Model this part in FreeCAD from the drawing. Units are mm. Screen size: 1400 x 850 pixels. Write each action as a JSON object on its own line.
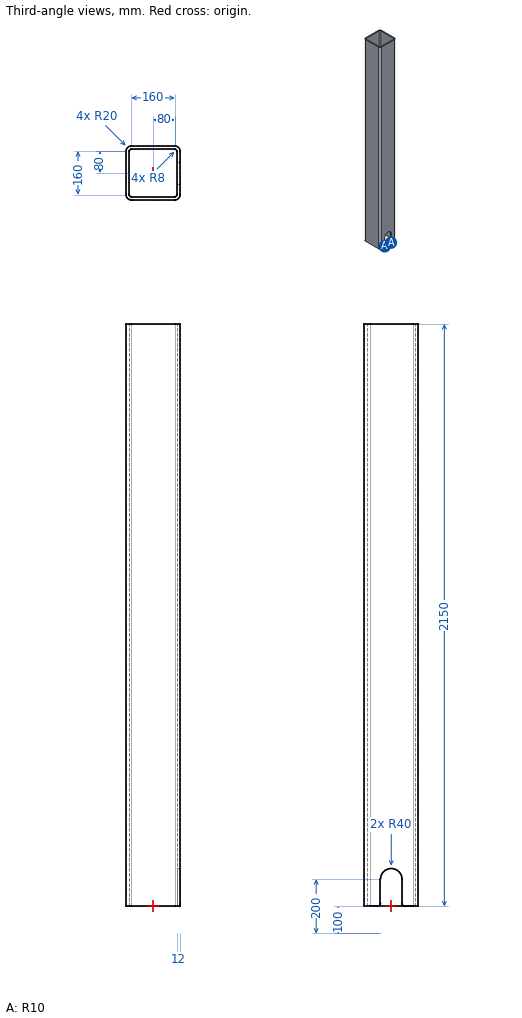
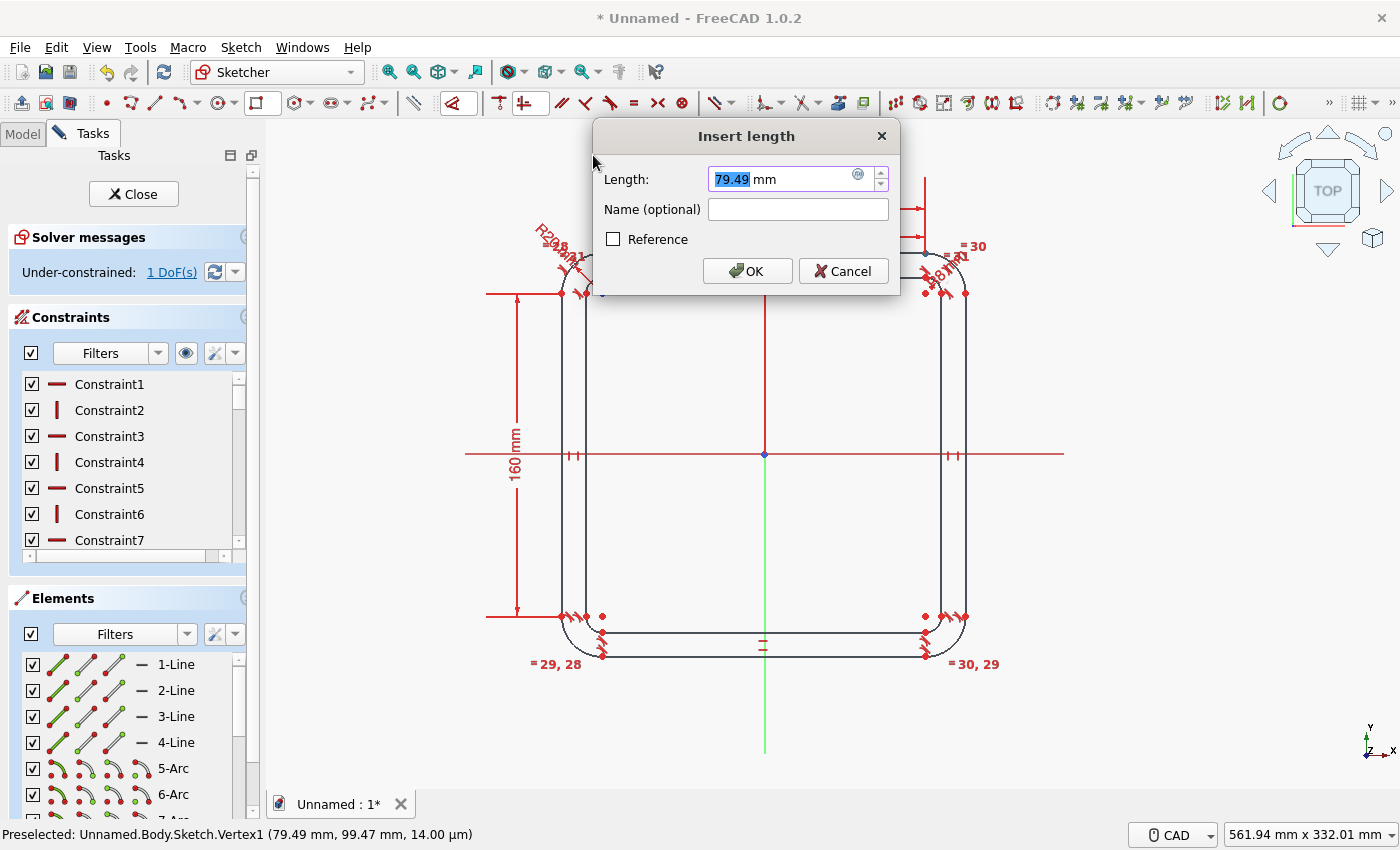
{"action": "type", "text": "80"}
{"action": "key", "text": "Return"}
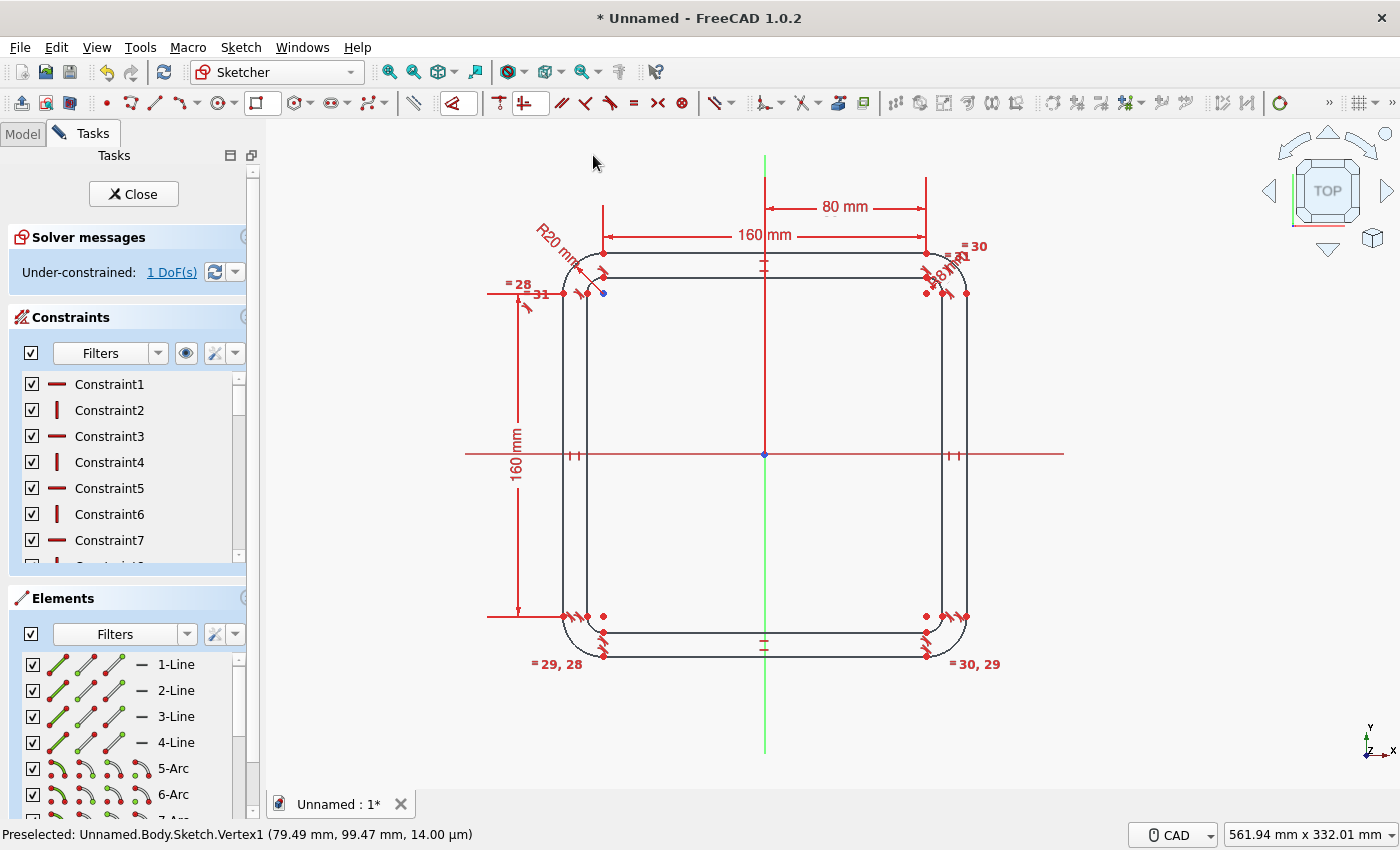
{"action": "left_click", "coordinate": [563, 294]}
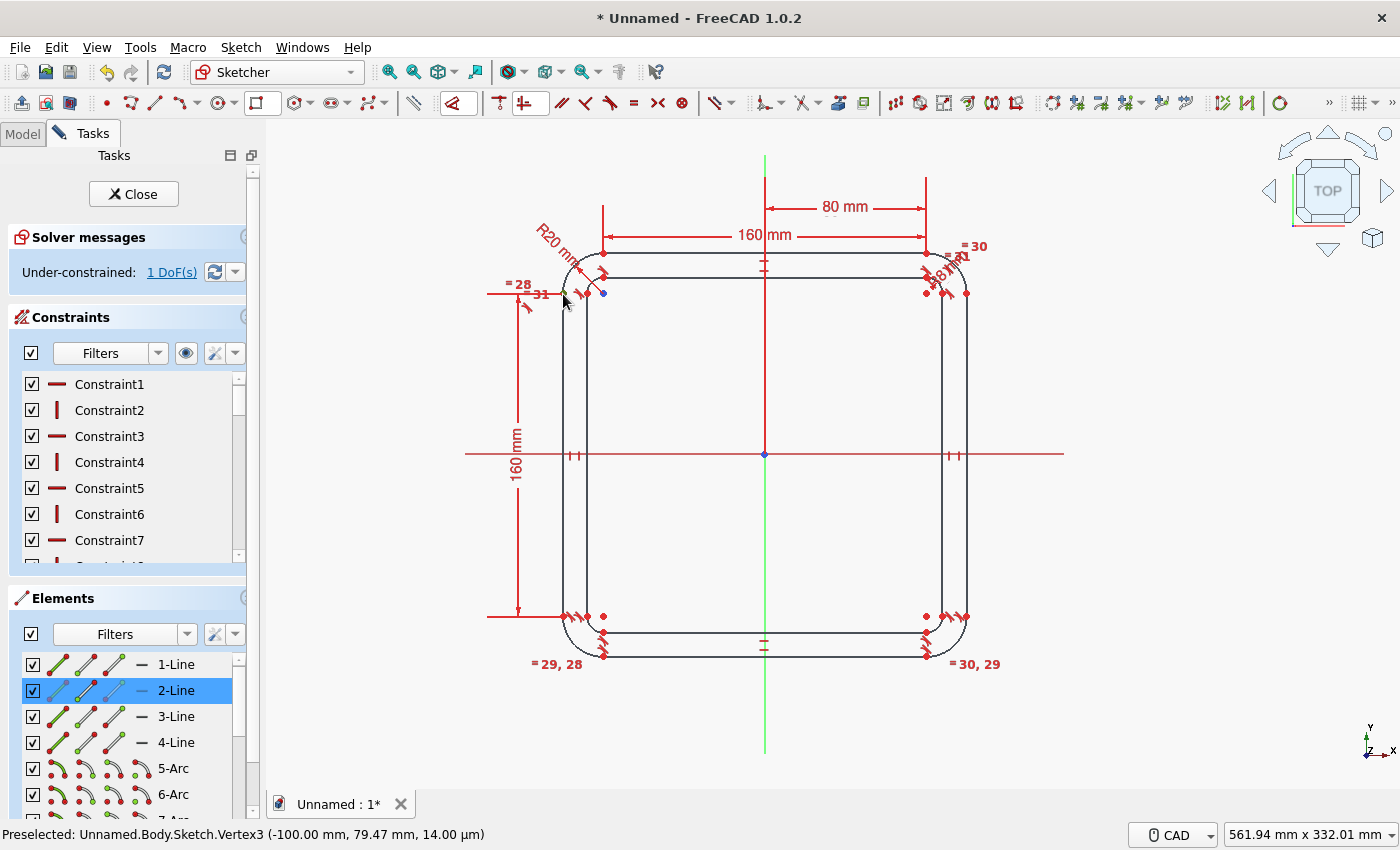
{"action": "left_click", "coordinate": [472, 104]}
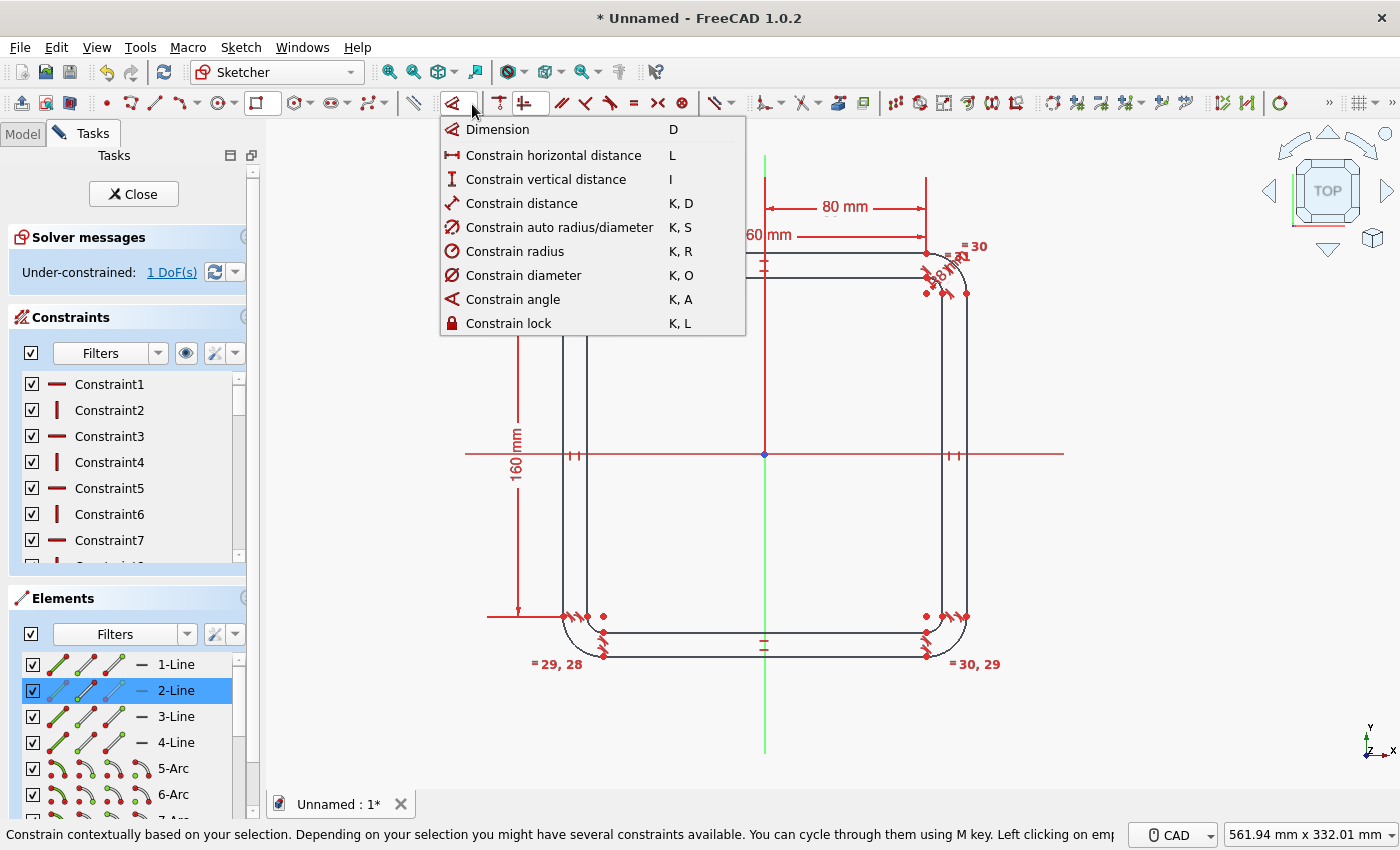
{"action": "left_click", "coordinate": [593, 179]}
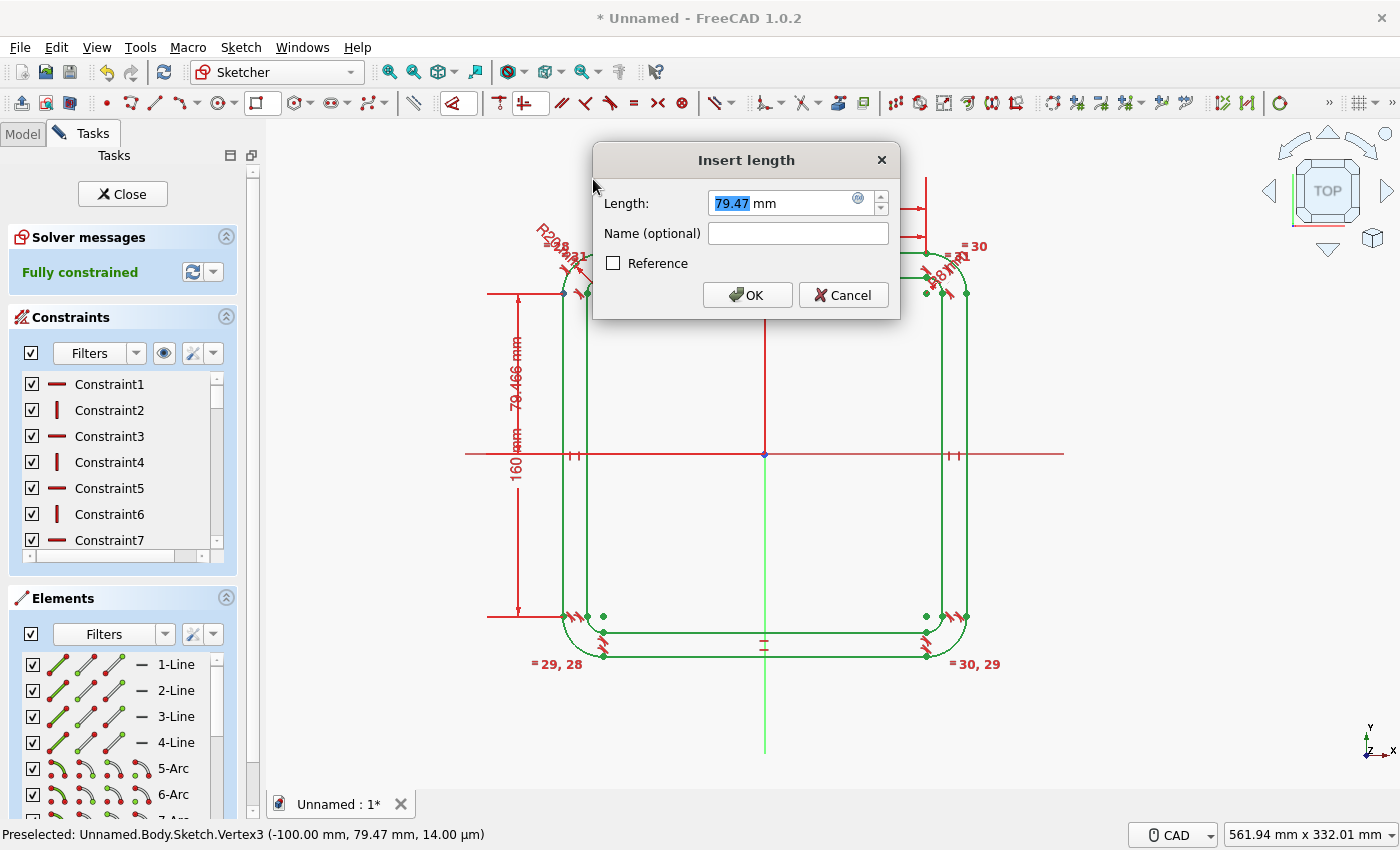
{"action": "type", "text": "80"}
{"action": "key", "text": "Return"}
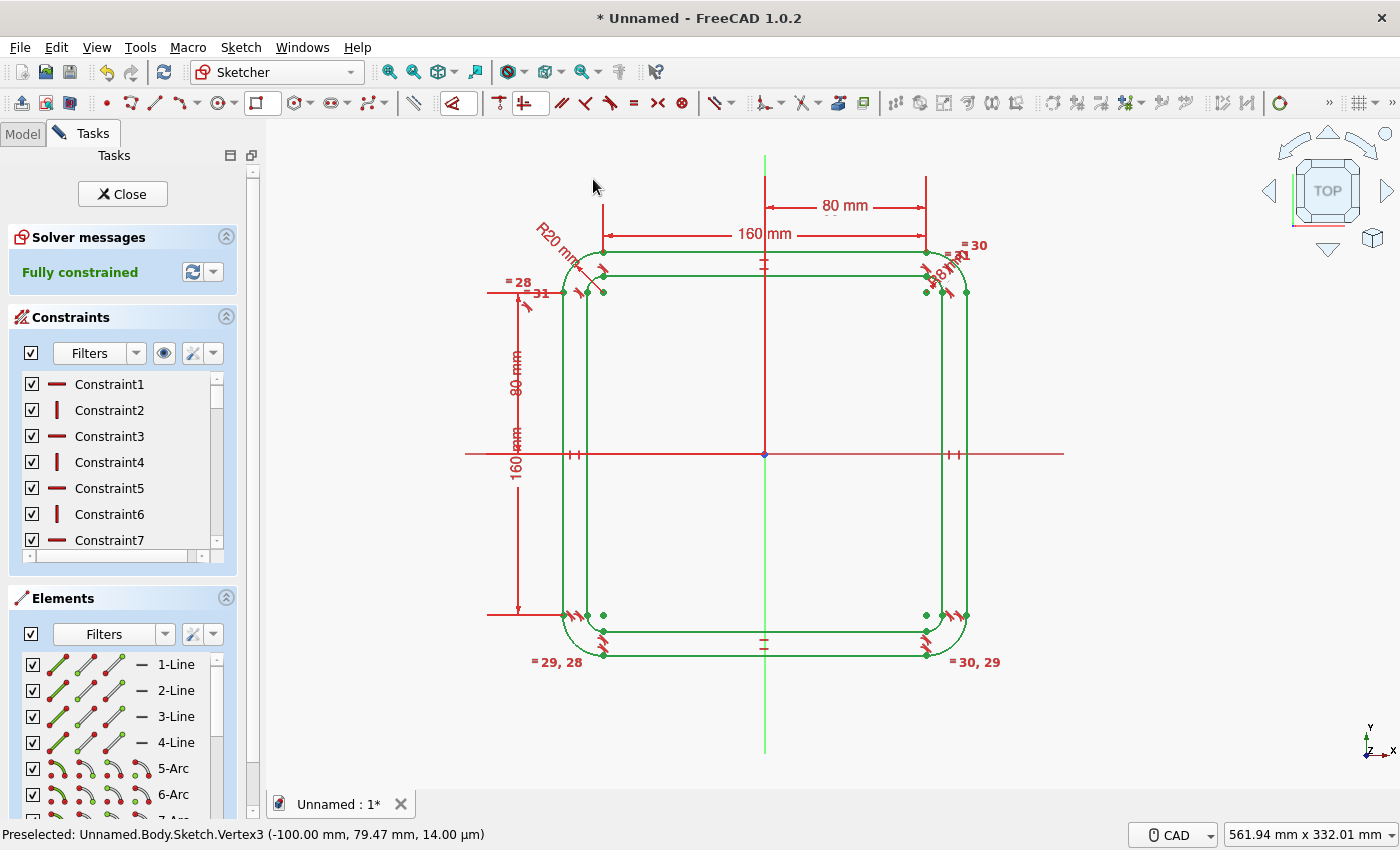
{"action": "left_click", "coordinate": [123, 194]}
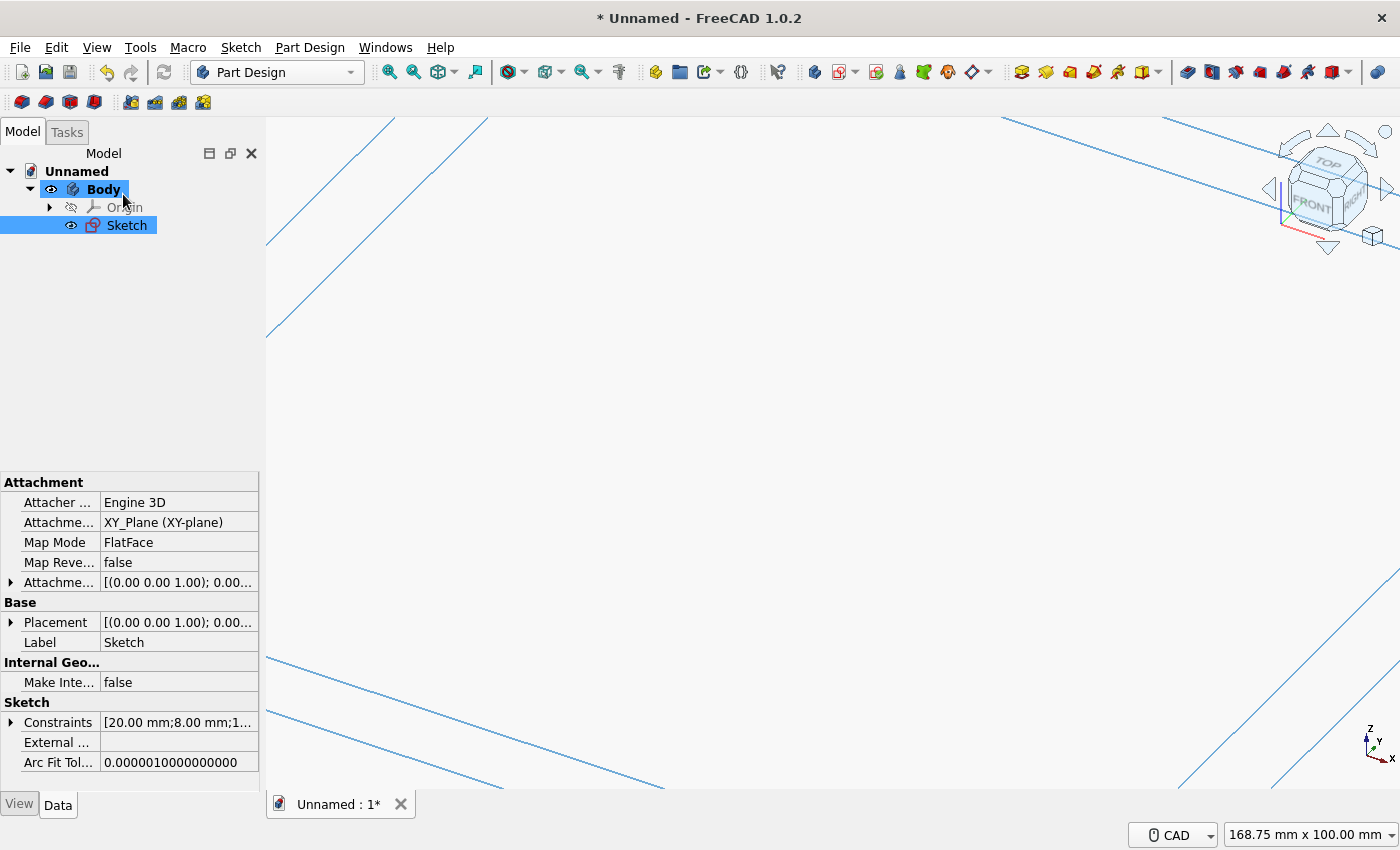
{"action": "left_click", "coordinate": [1022, 72]}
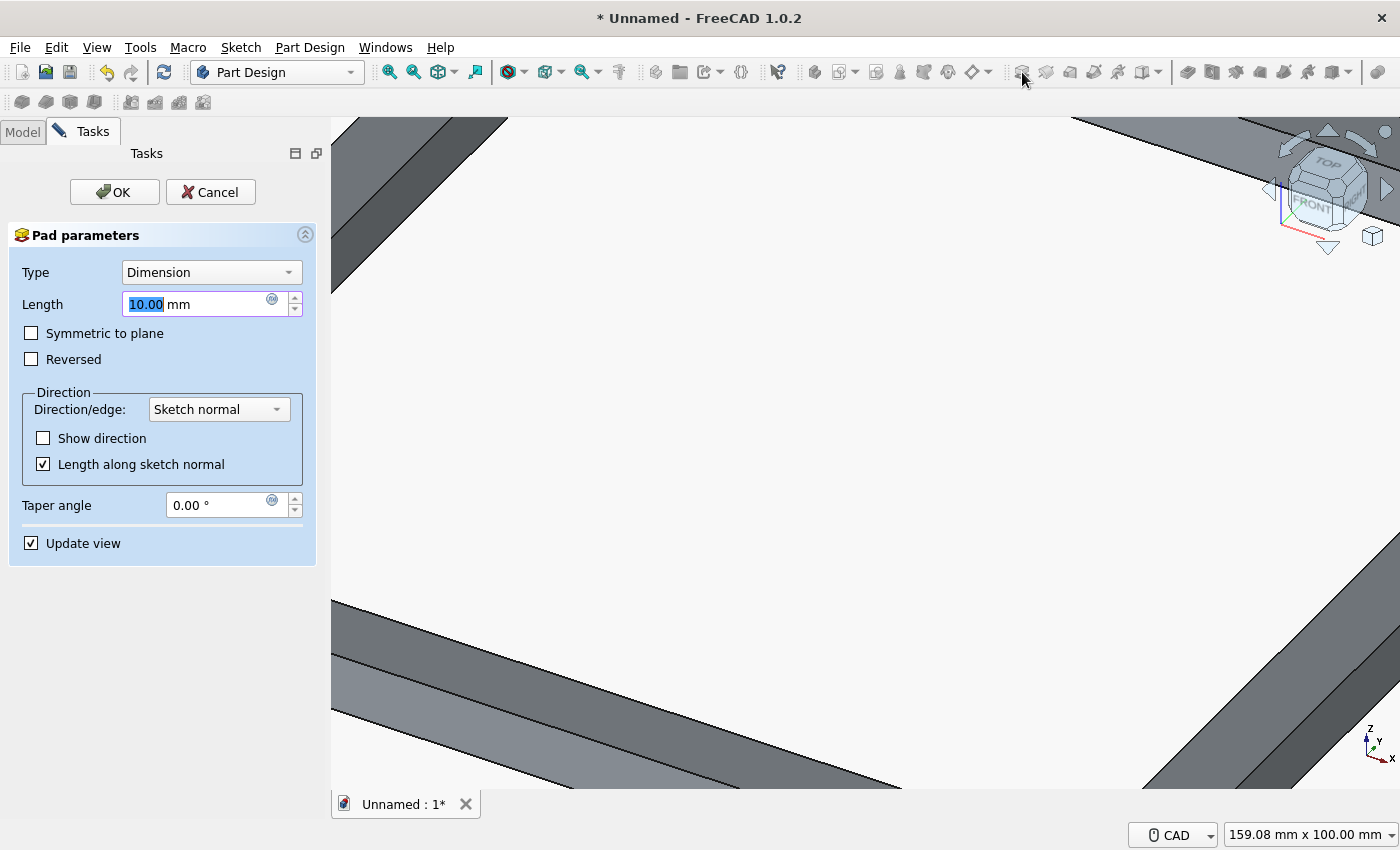
{"action": "type", "text": "2150"}
{"action": "key", "text": "Tab"}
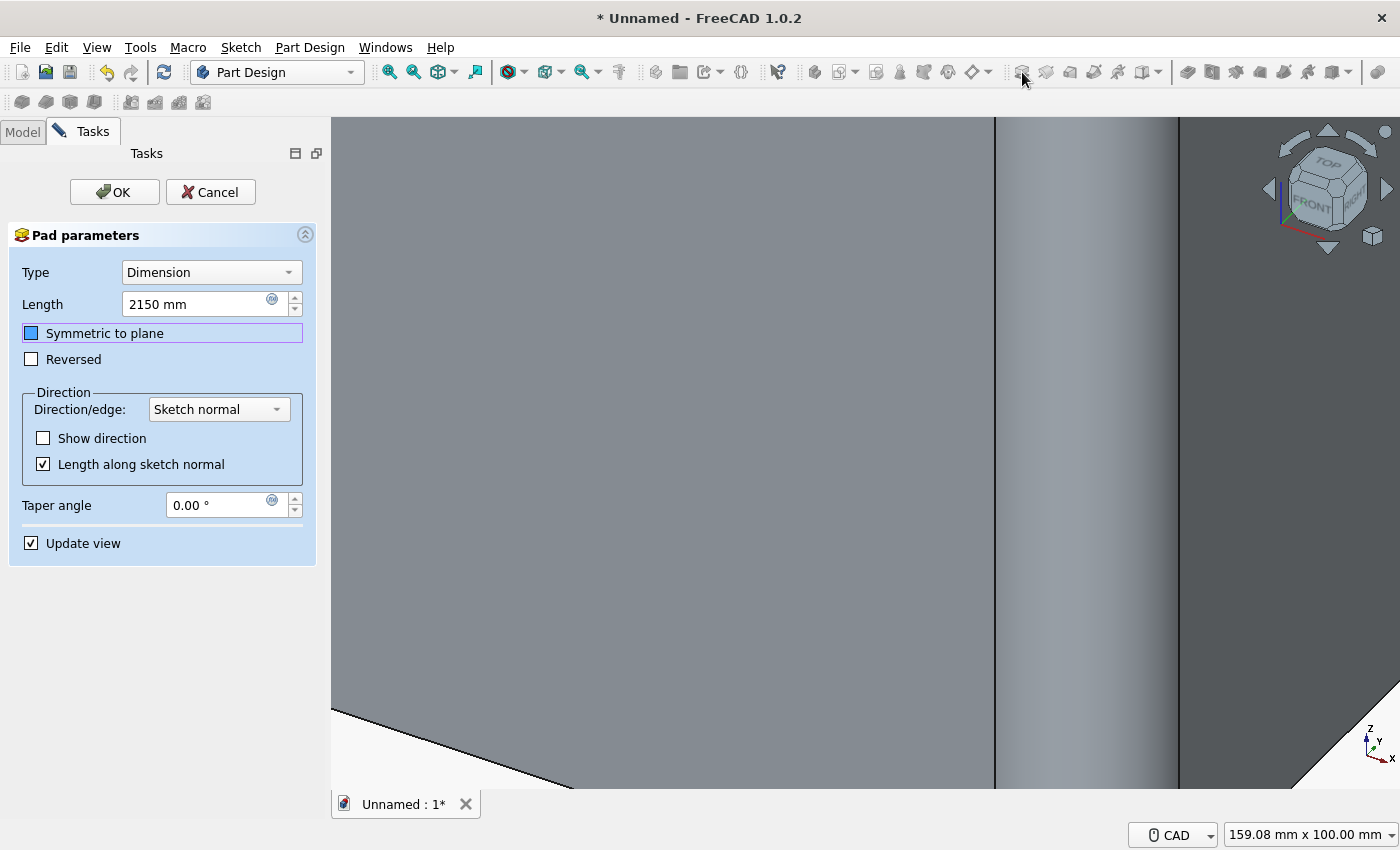
{"action": "left_click", "coordinate": [115, 192]}